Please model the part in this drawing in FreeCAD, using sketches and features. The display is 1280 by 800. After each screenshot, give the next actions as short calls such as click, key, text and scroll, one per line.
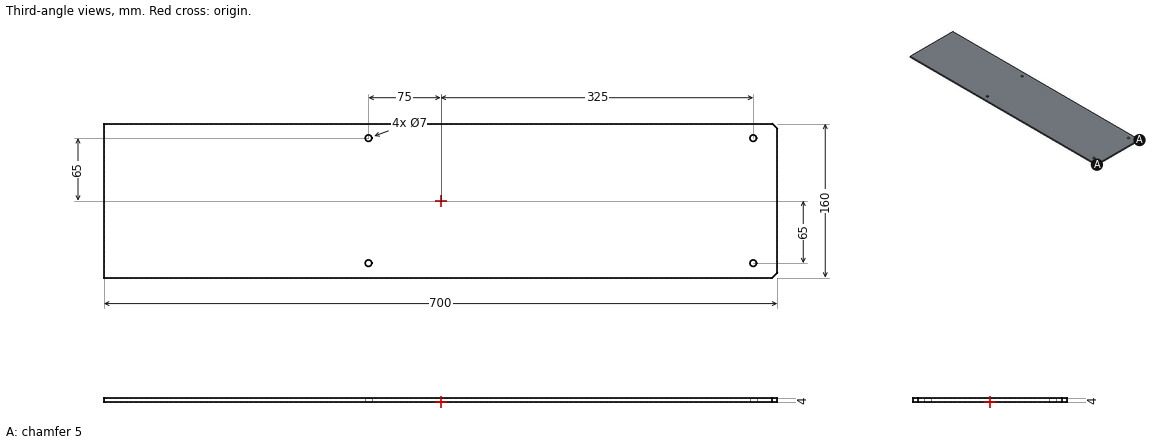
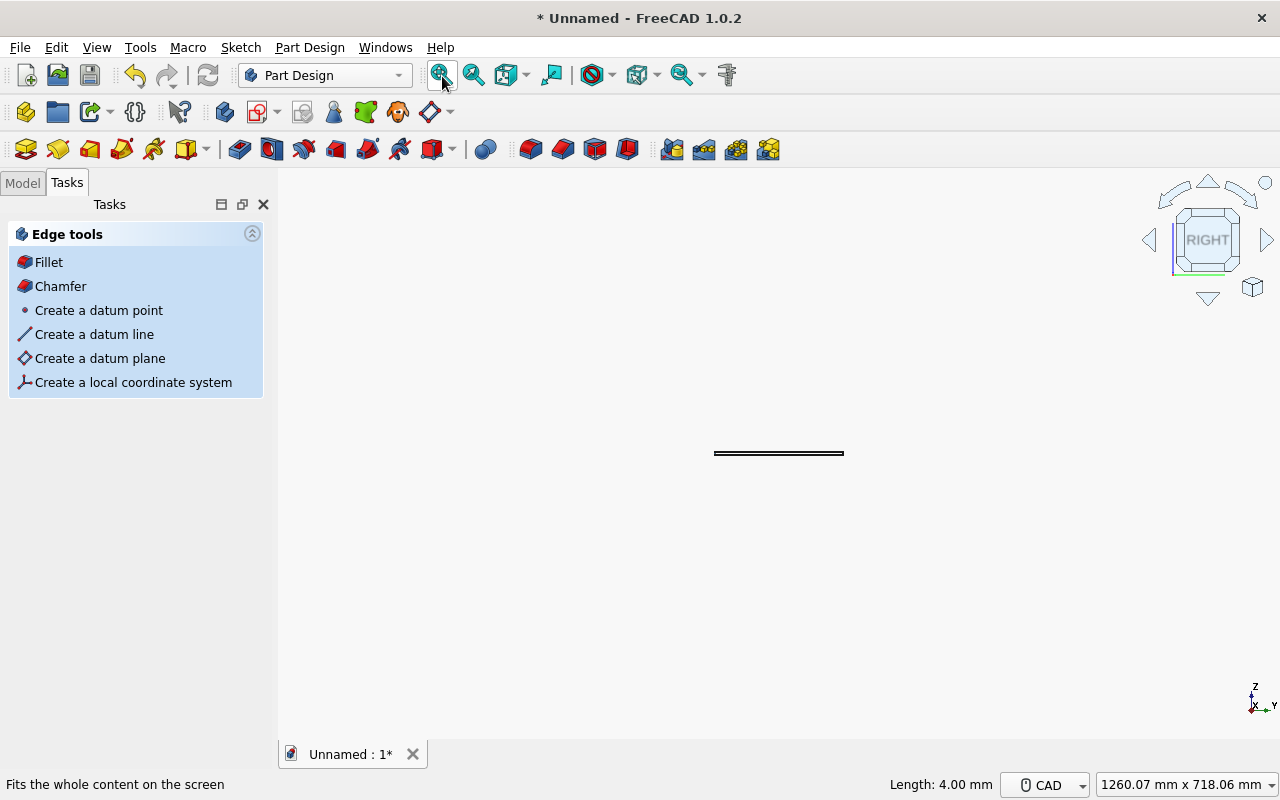
scroll(843, 452, up, 13)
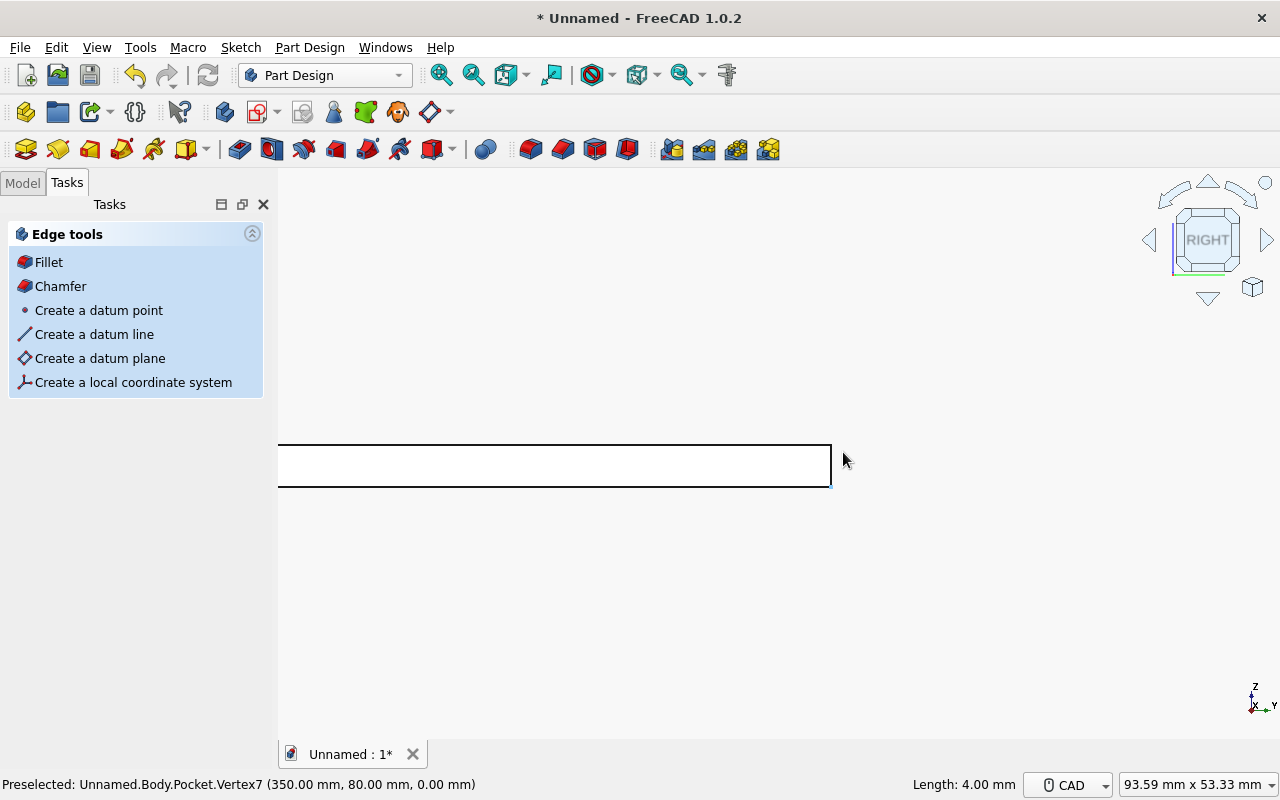
click(831, 465, ctrl)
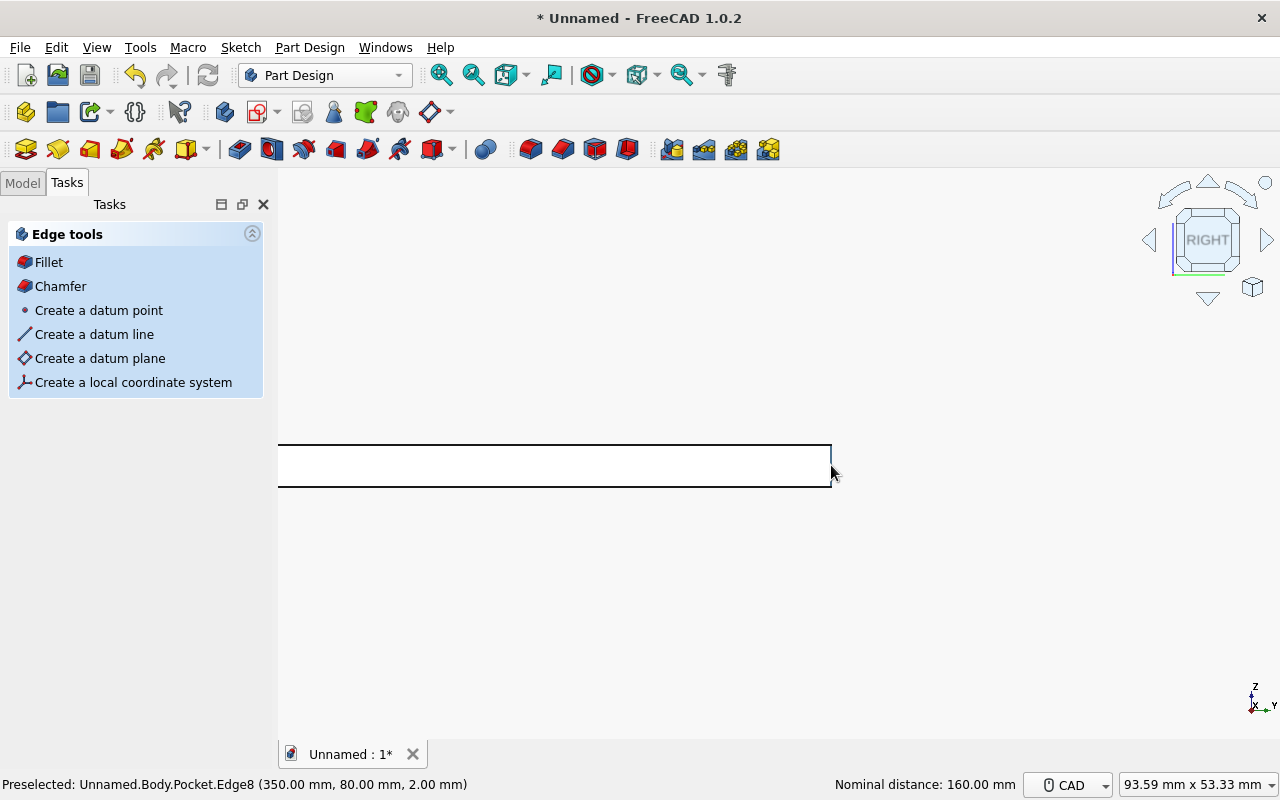
click(564, 150)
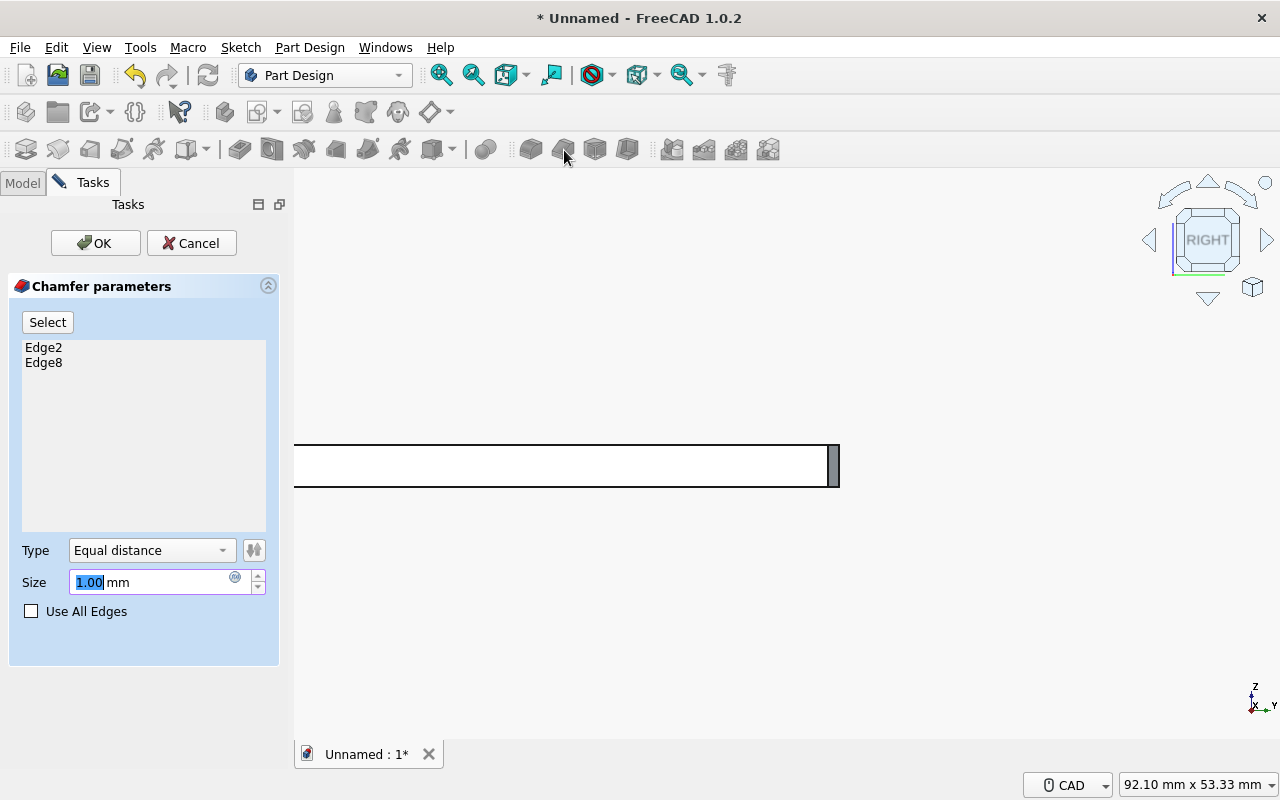
text(5)
key(Tab)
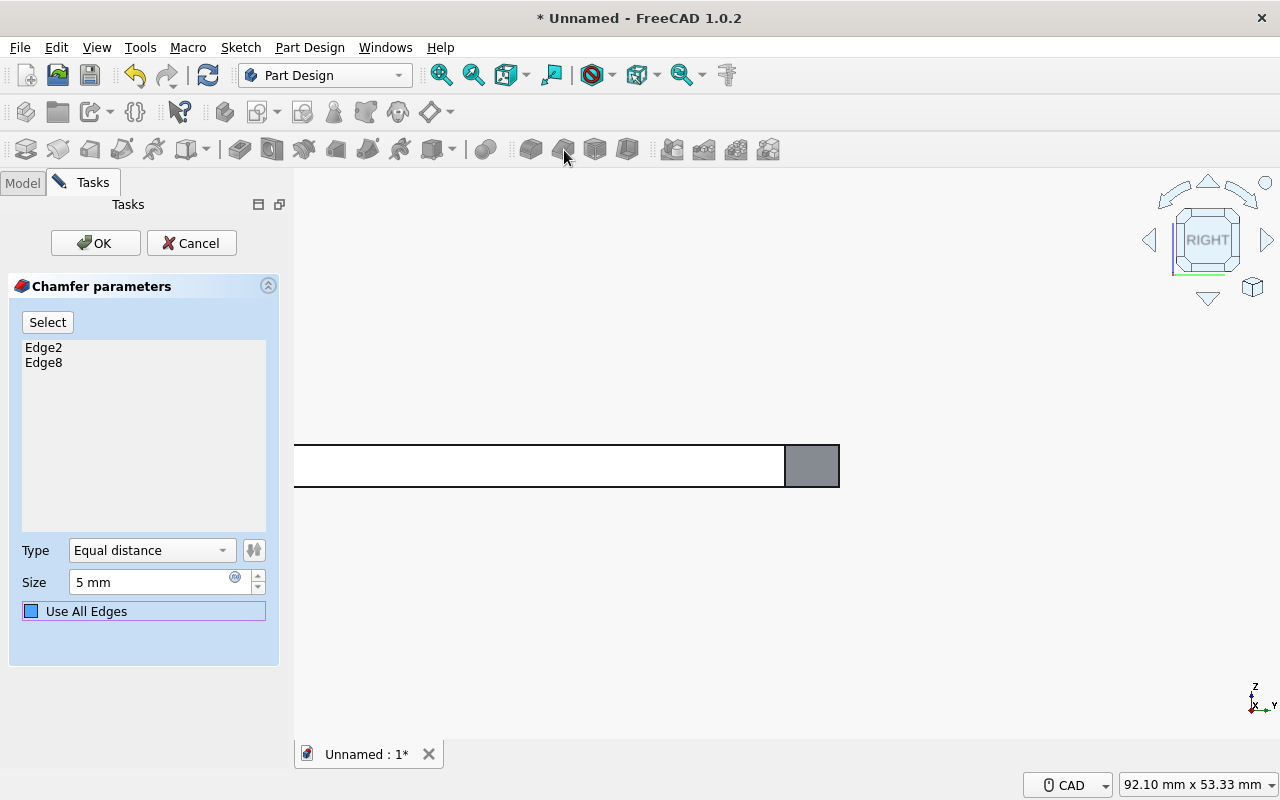
click(96, 243)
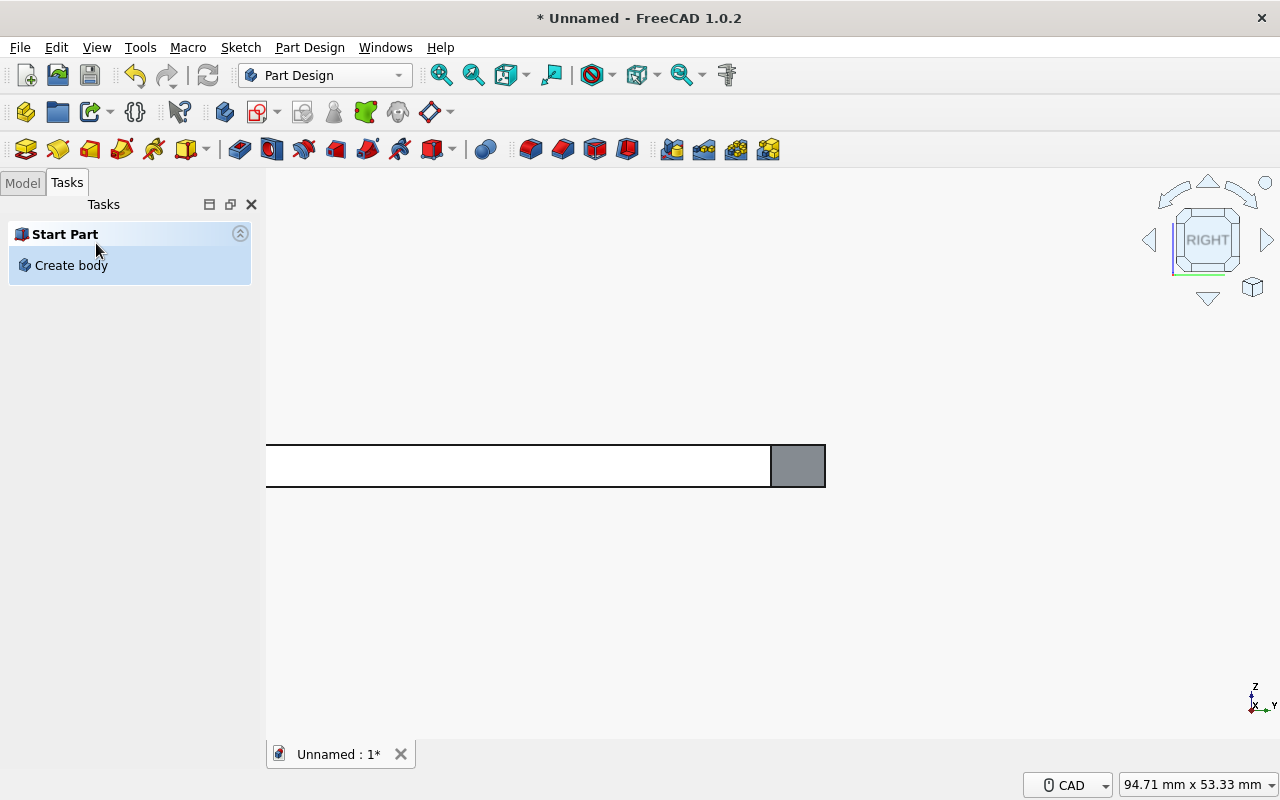
key(0)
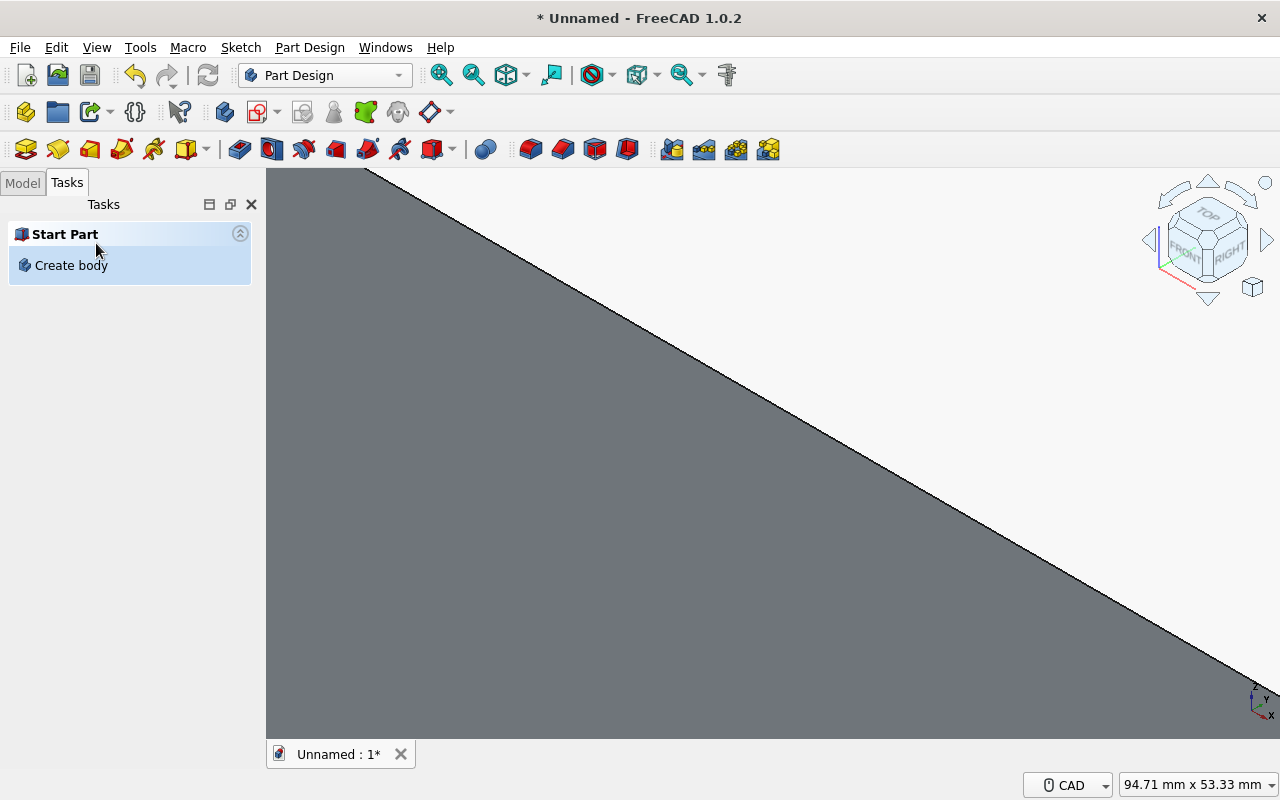
click(442, 76)